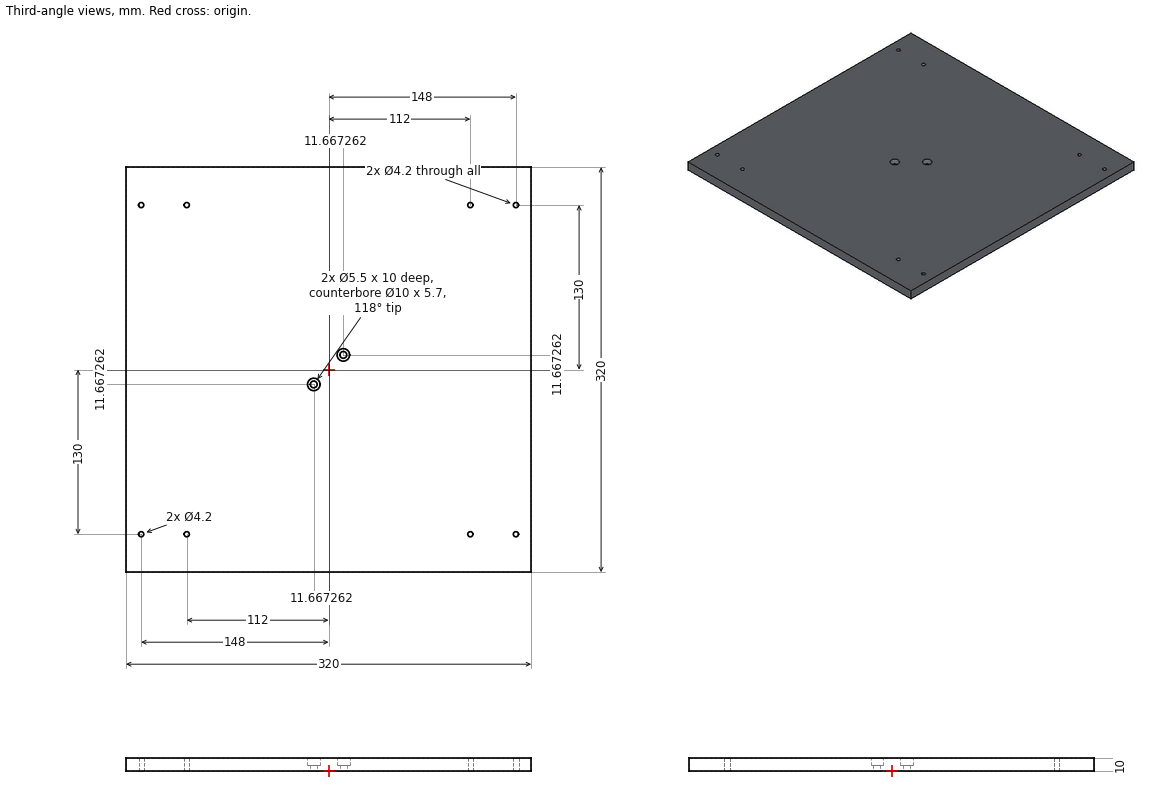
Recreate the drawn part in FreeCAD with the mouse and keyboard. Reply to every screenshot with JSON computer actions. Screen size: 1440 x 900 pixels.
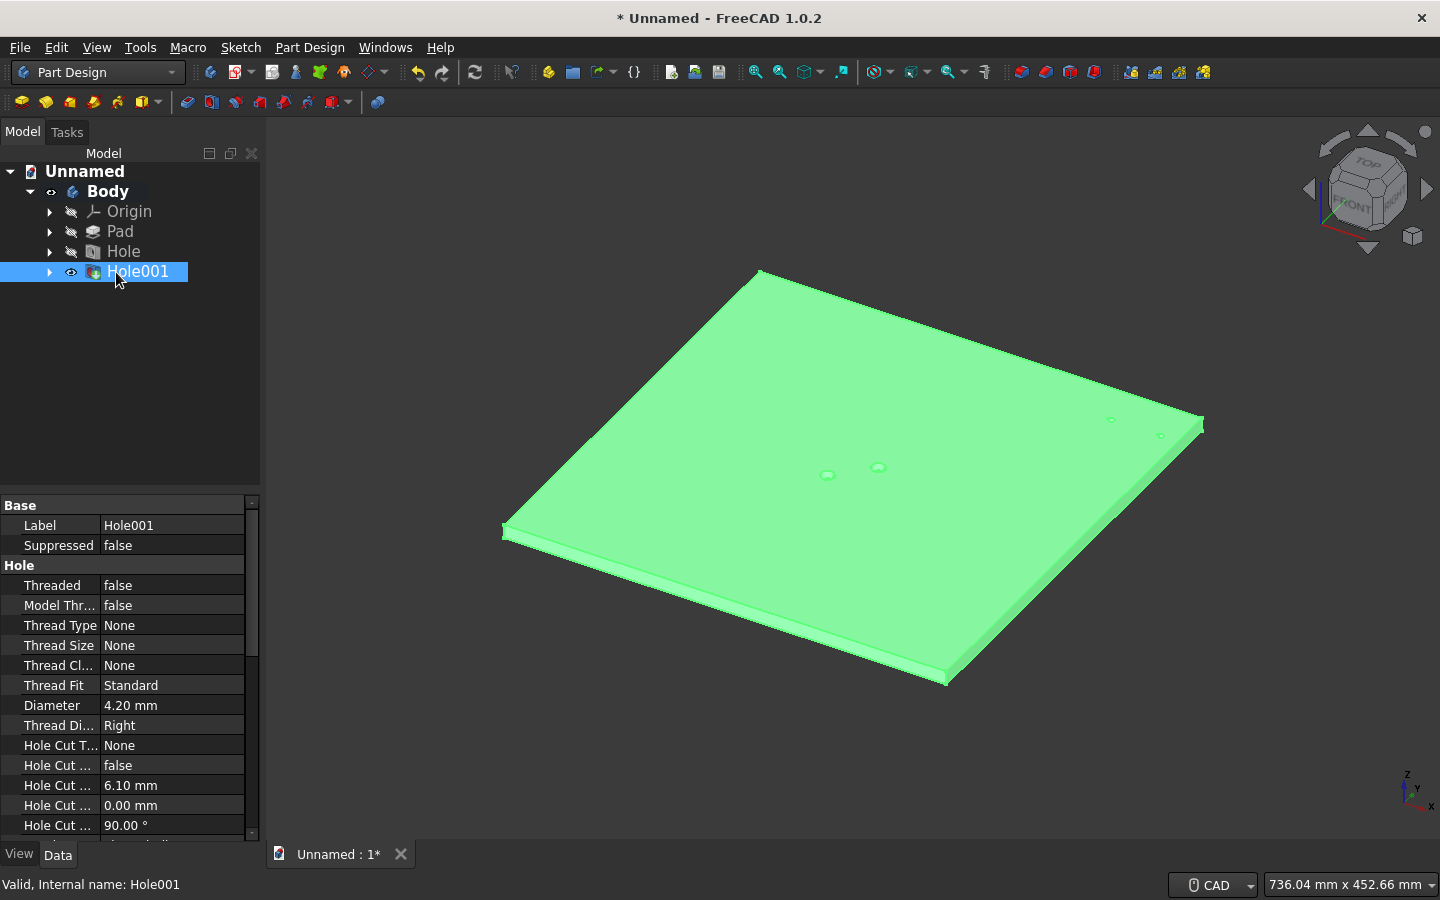
{"action": "left_click", "coordinate": [1132, 72]}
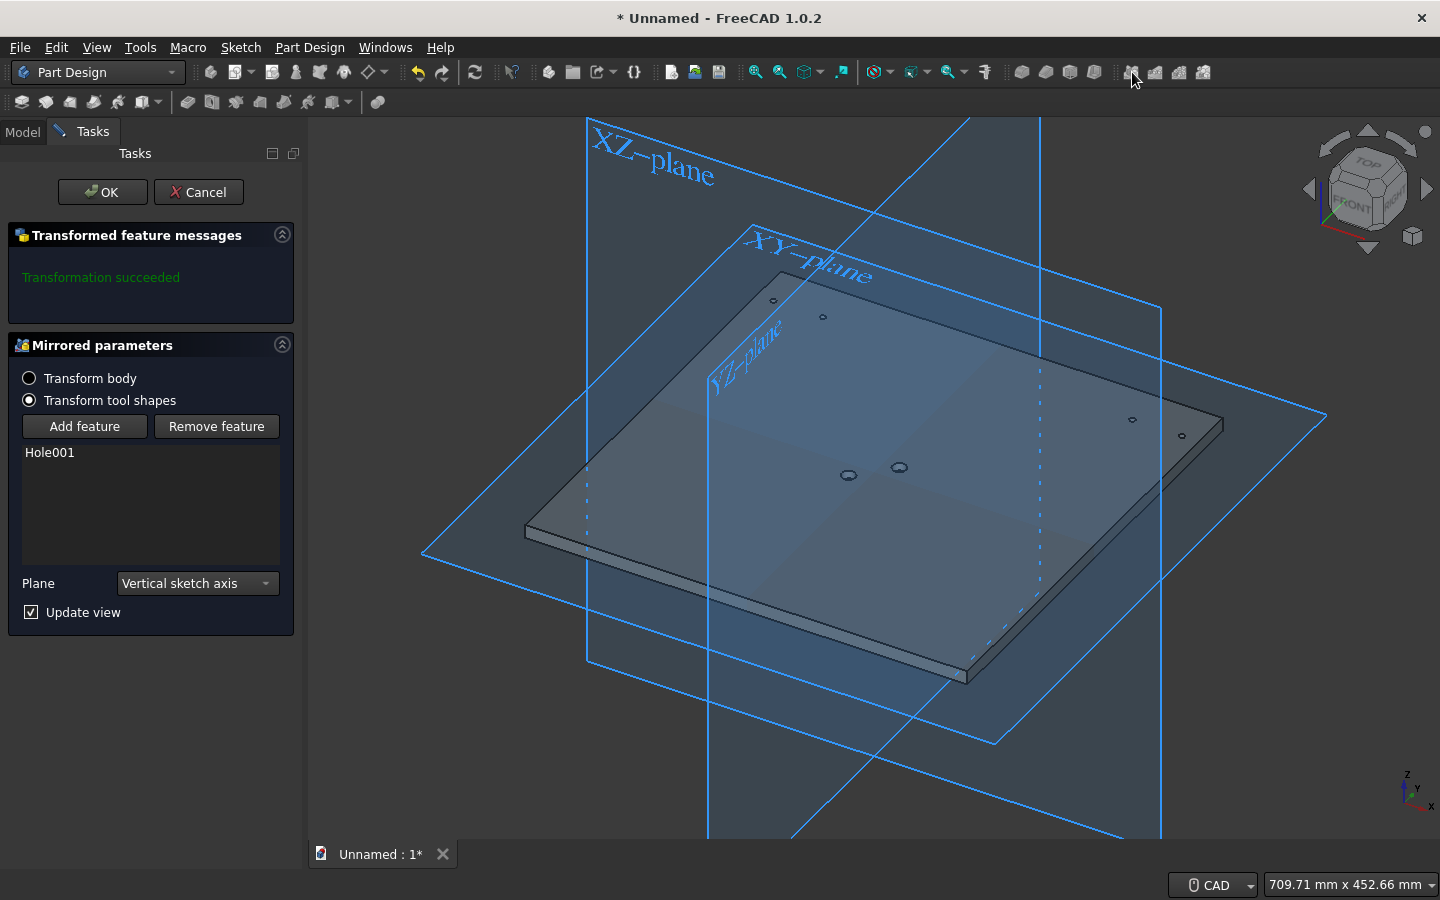
{"action": "left_click", "coordinate": [198, 584]}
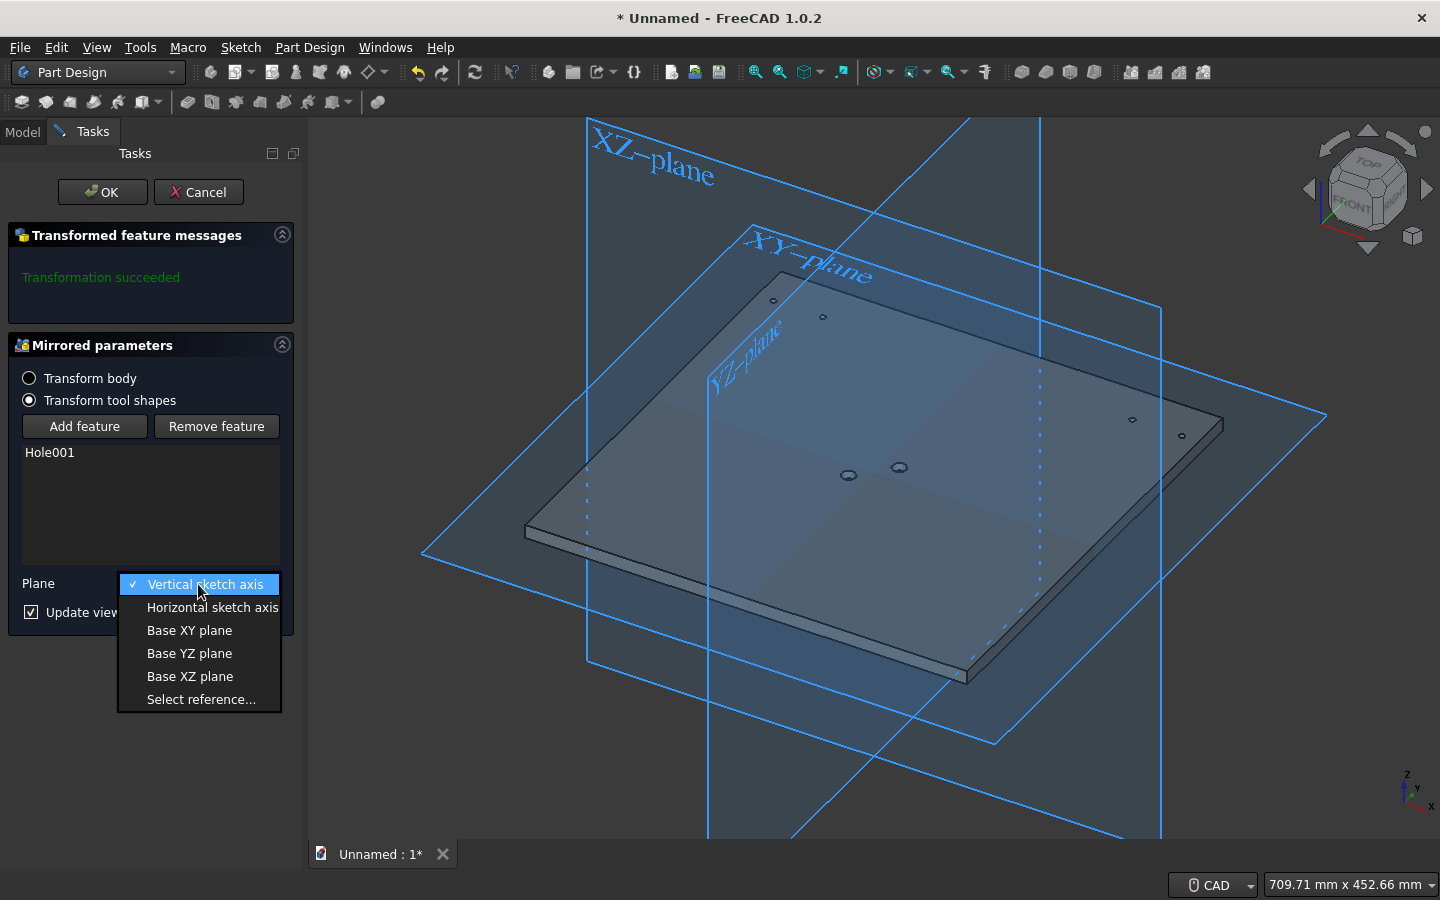
{"action": "left_click", "coordinate": [198, 676]}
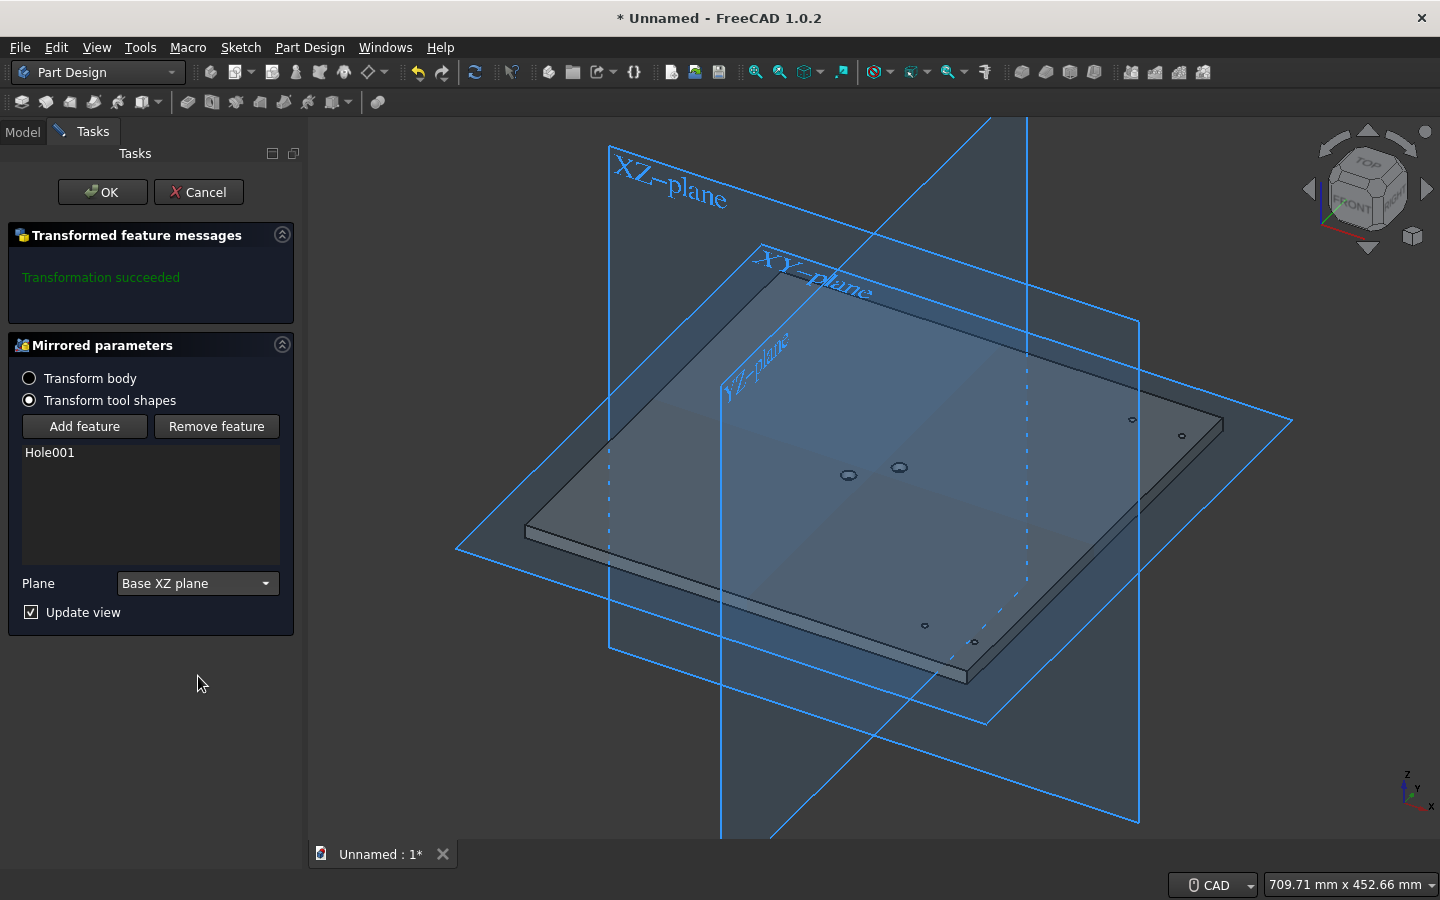
{"action": "left_click", "coordinate": [103, 192]}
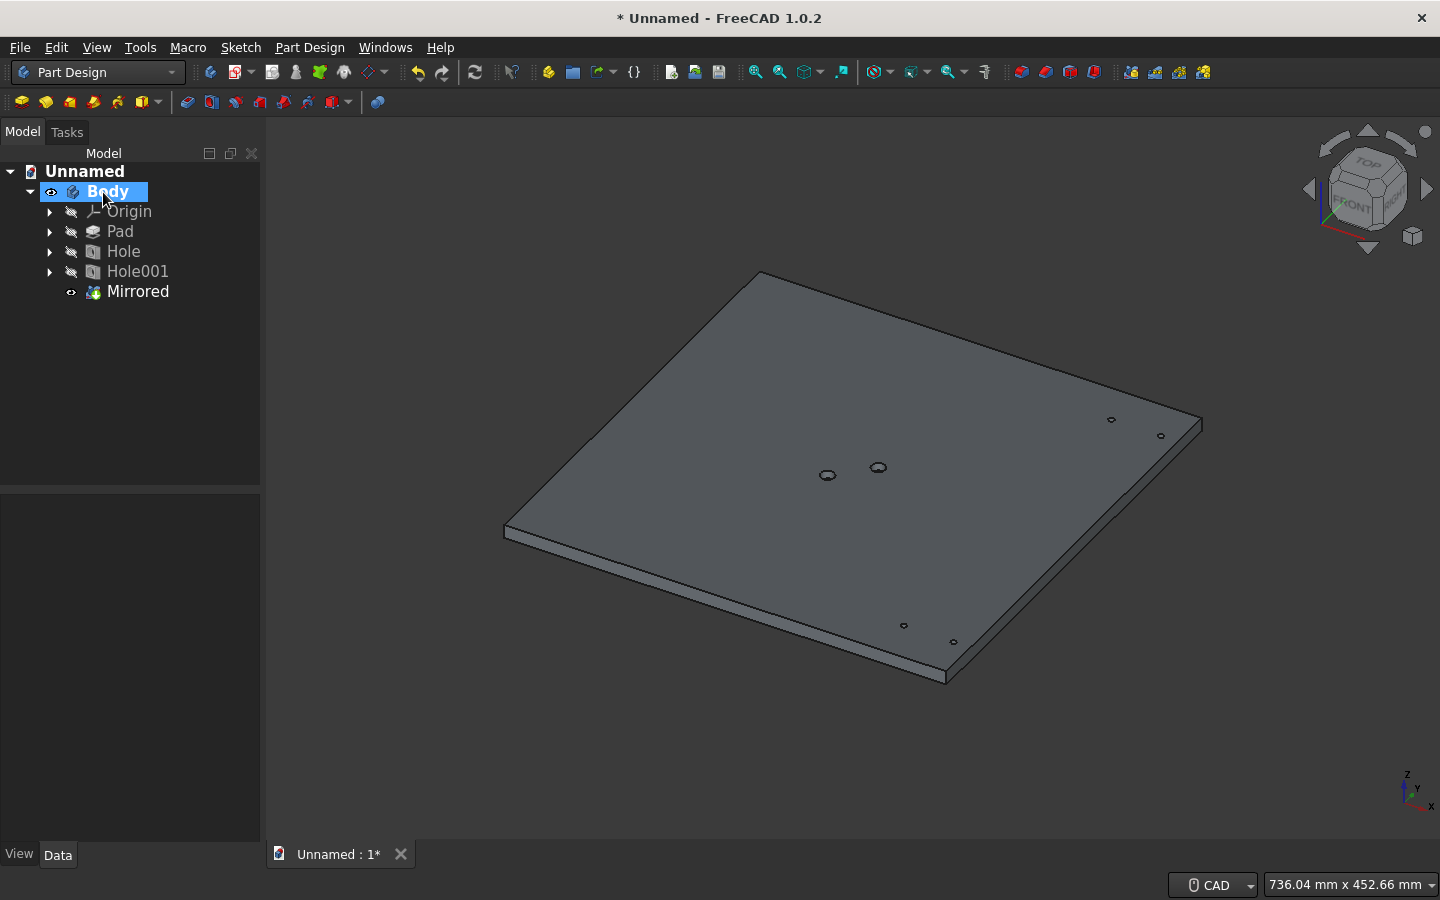
{"action": "left_click", "coordinate": [116, 272]}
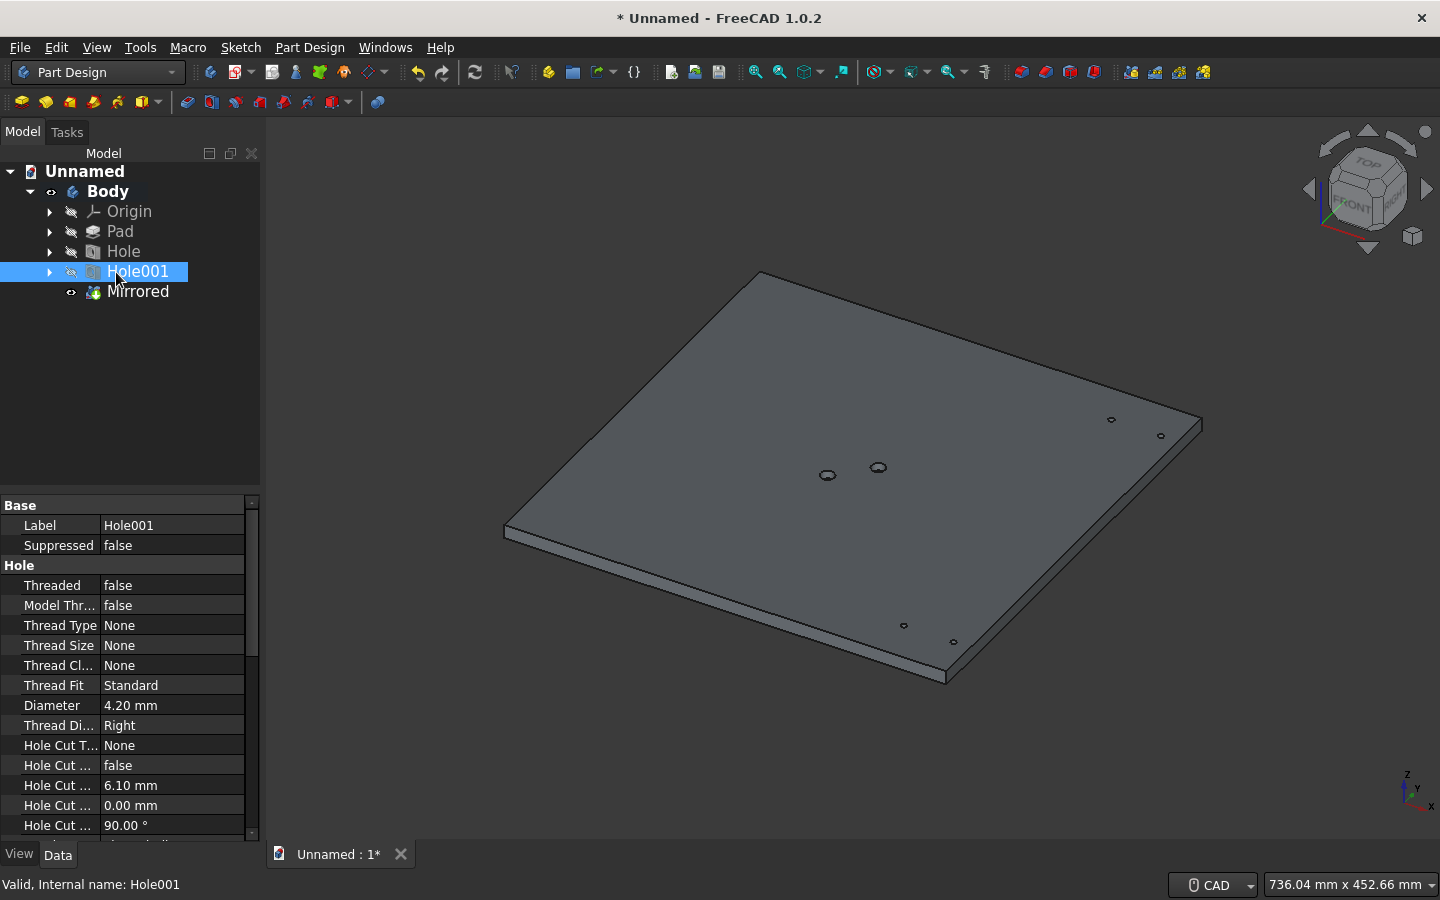
{"action": "left_click", "coordinate": [1132, 72]}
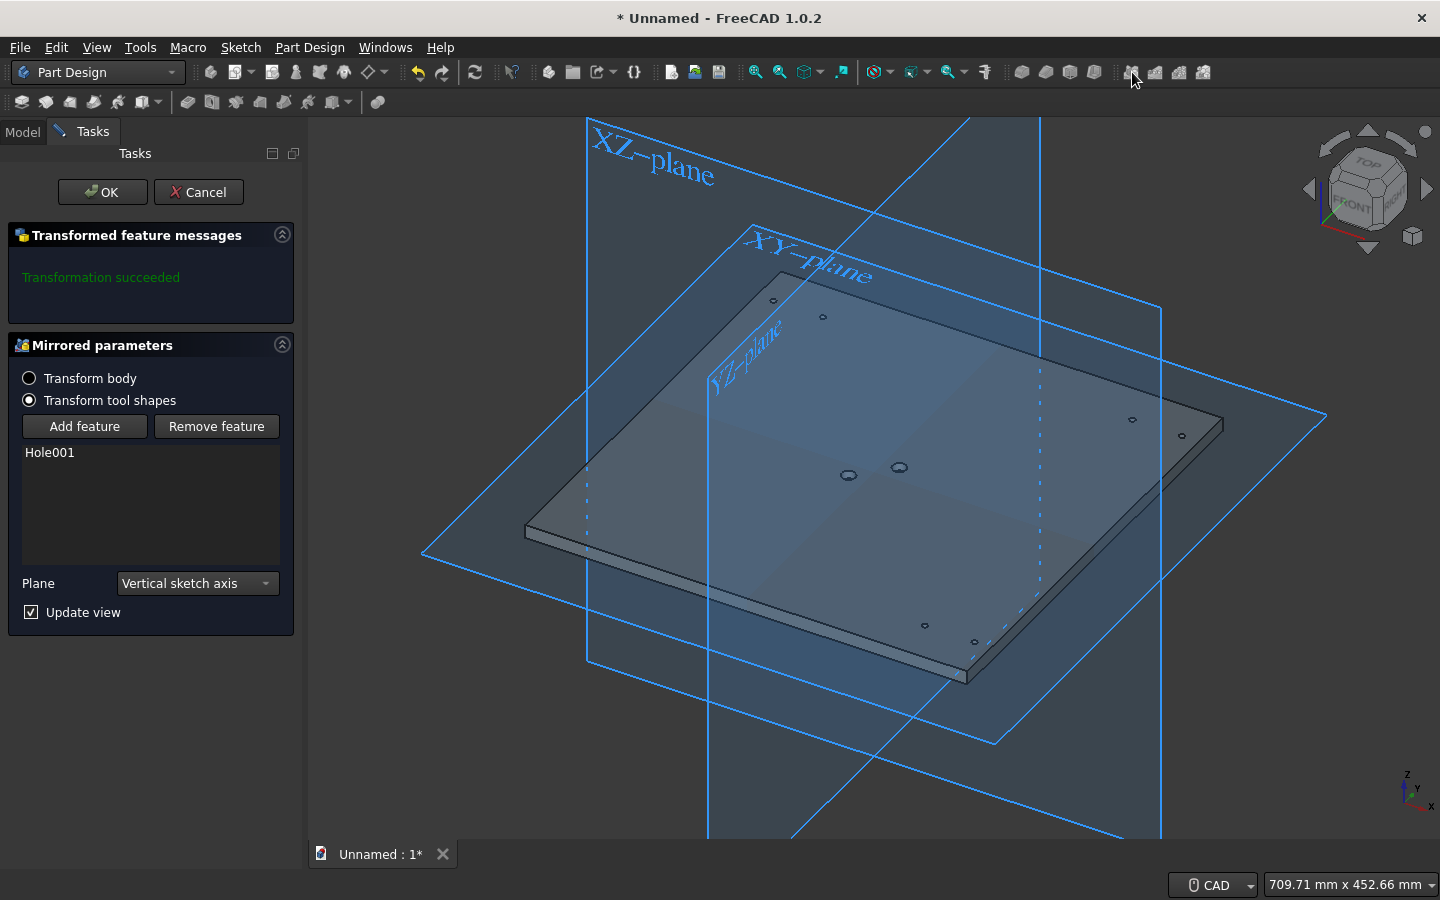
{"action": "left_click", "coordinate": [198, 584]}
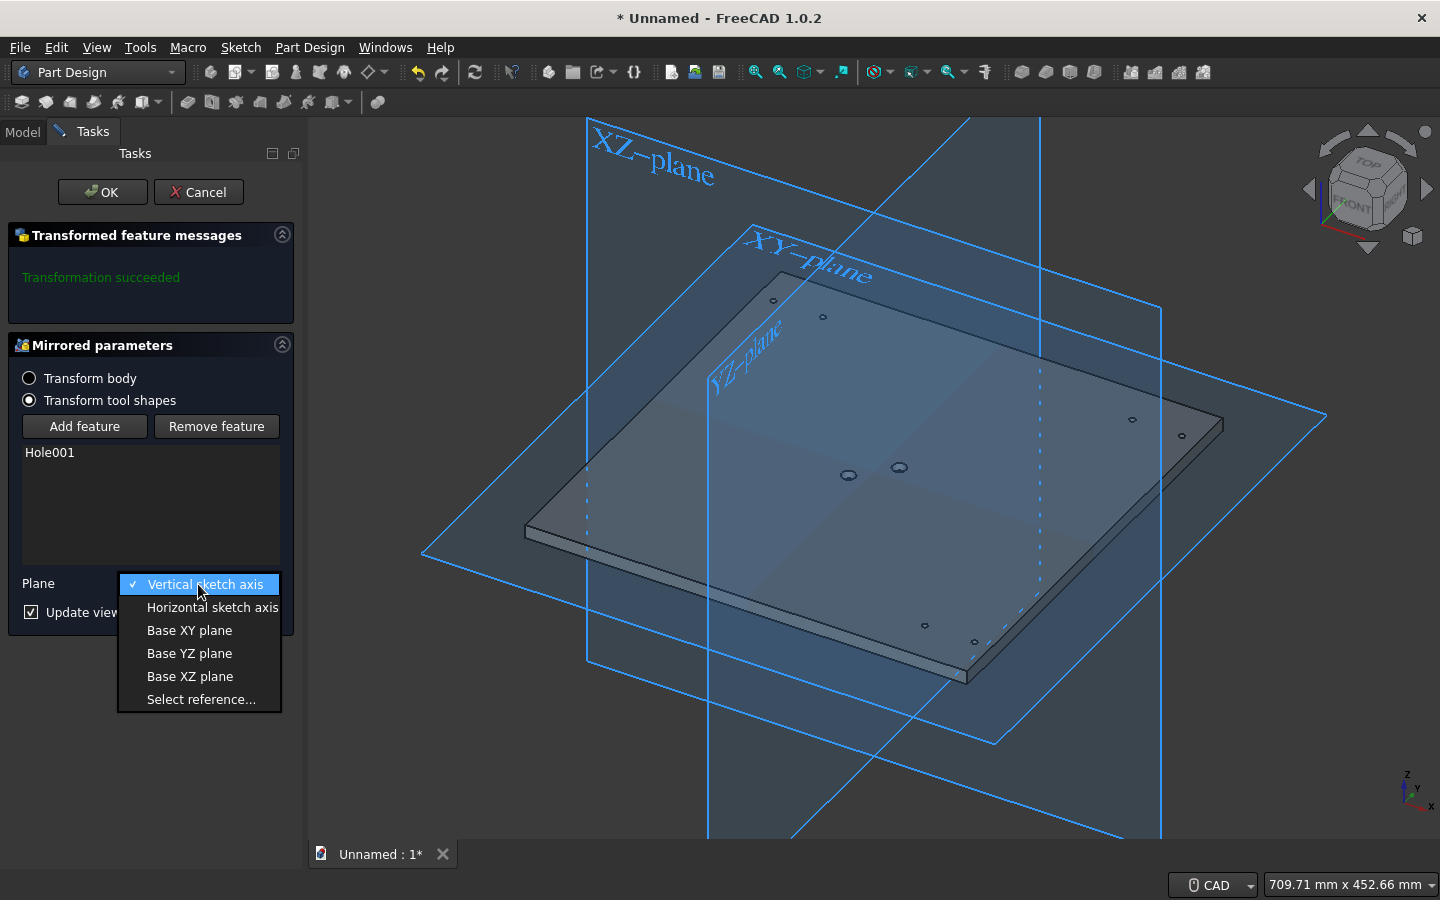
{"action": "left_click", "coordinate": [198, 654]}